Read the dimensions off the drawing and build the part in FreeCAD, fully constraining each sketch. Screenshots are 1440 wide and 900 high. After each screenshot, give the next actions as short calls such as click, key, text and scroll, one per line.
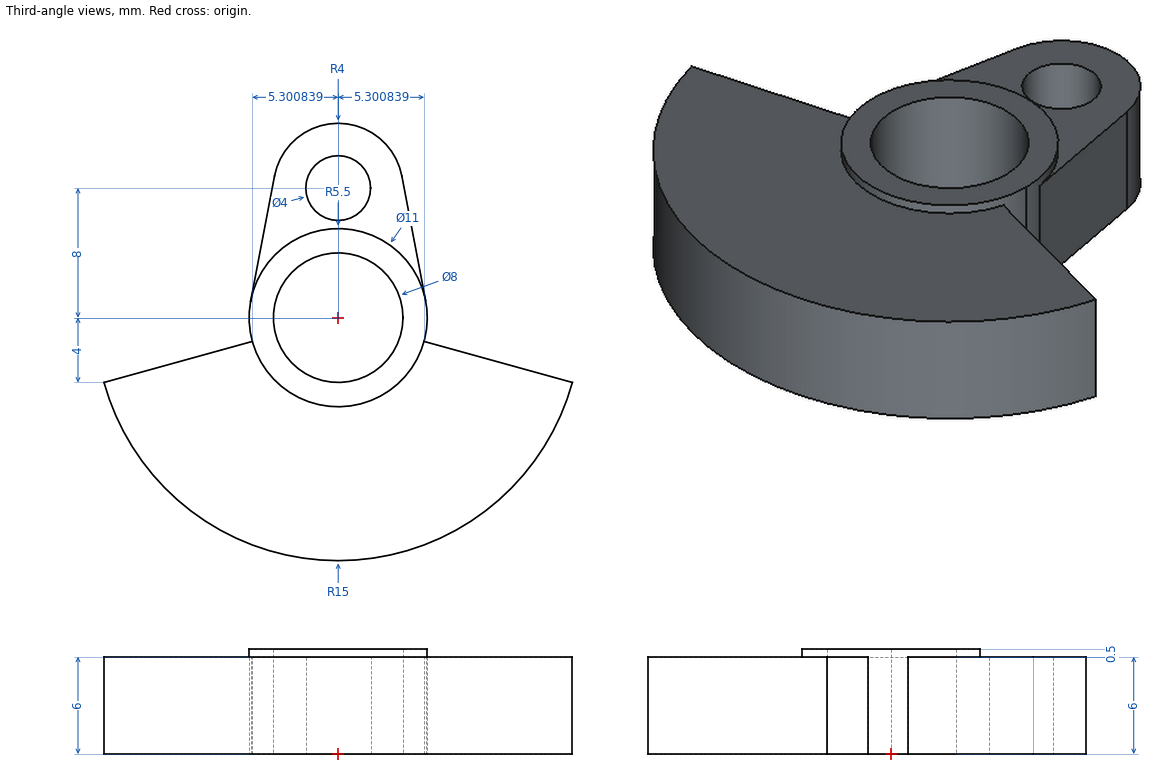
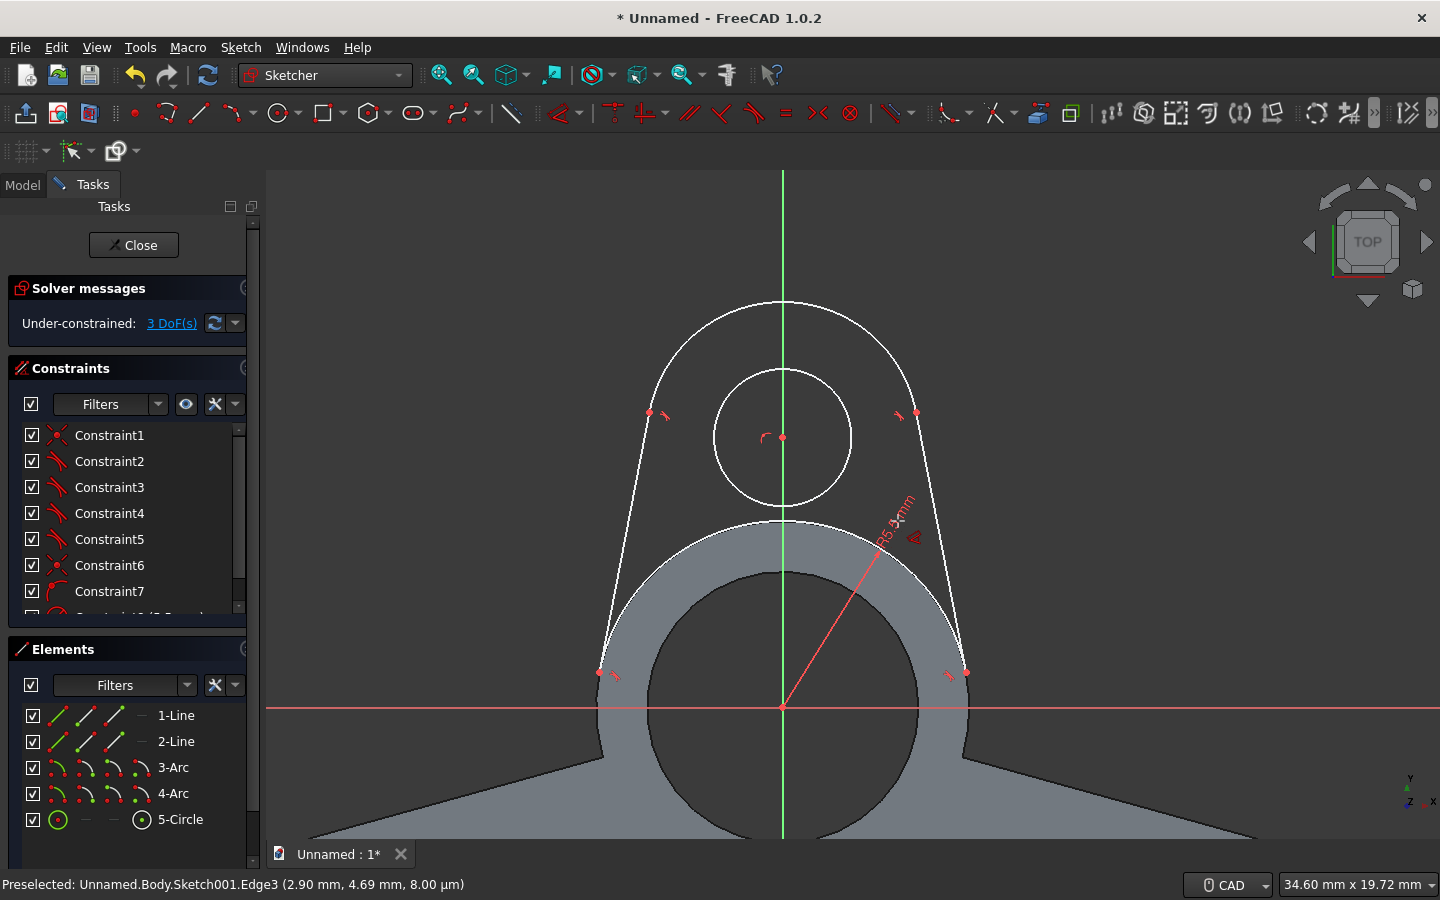
click(854, 322)
click(871, 295)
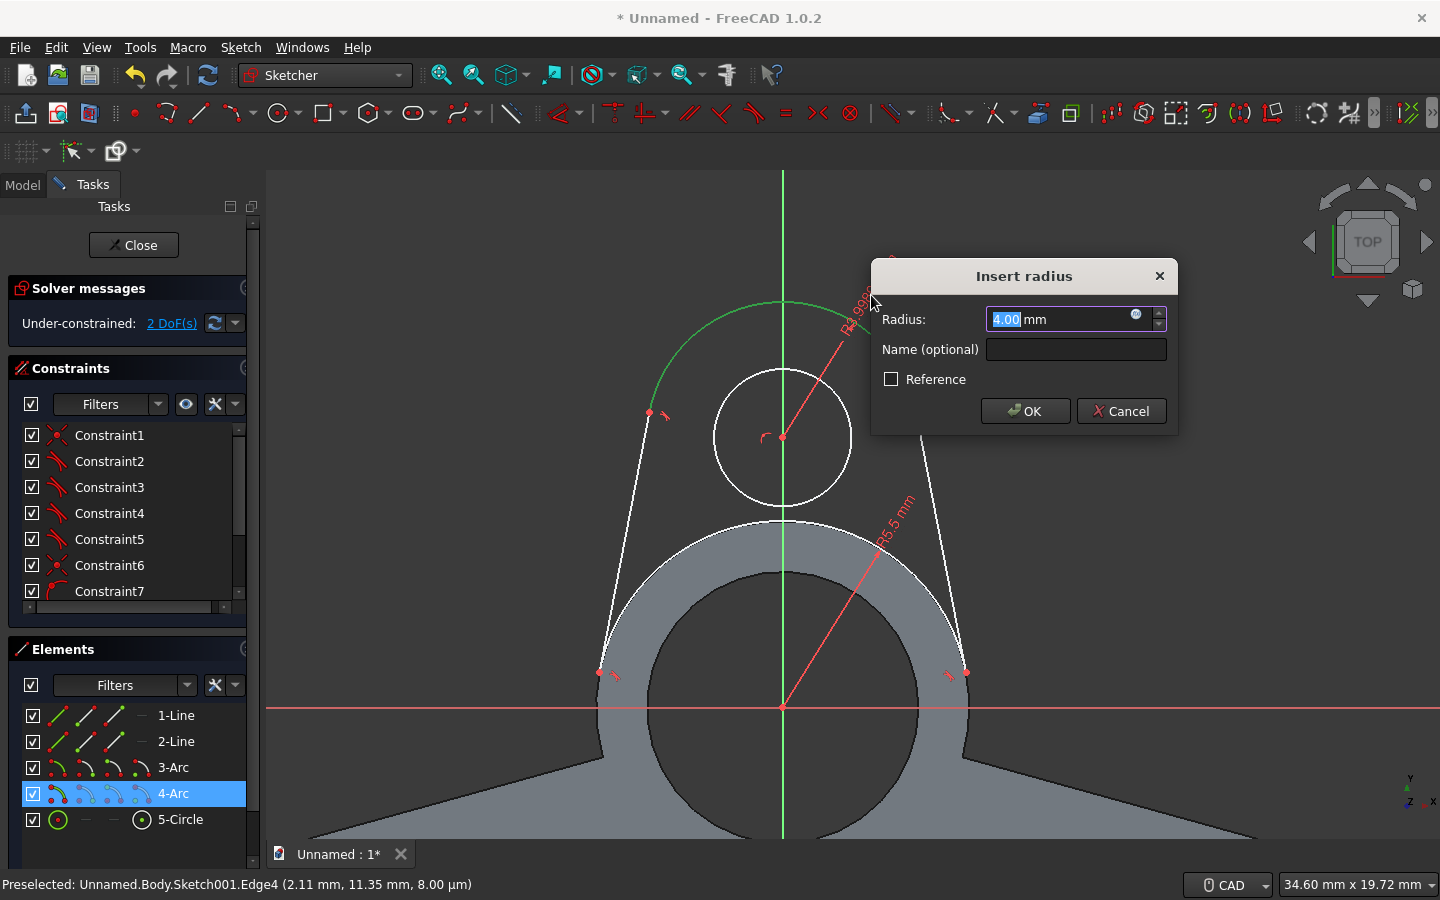
text(4)
key(Return)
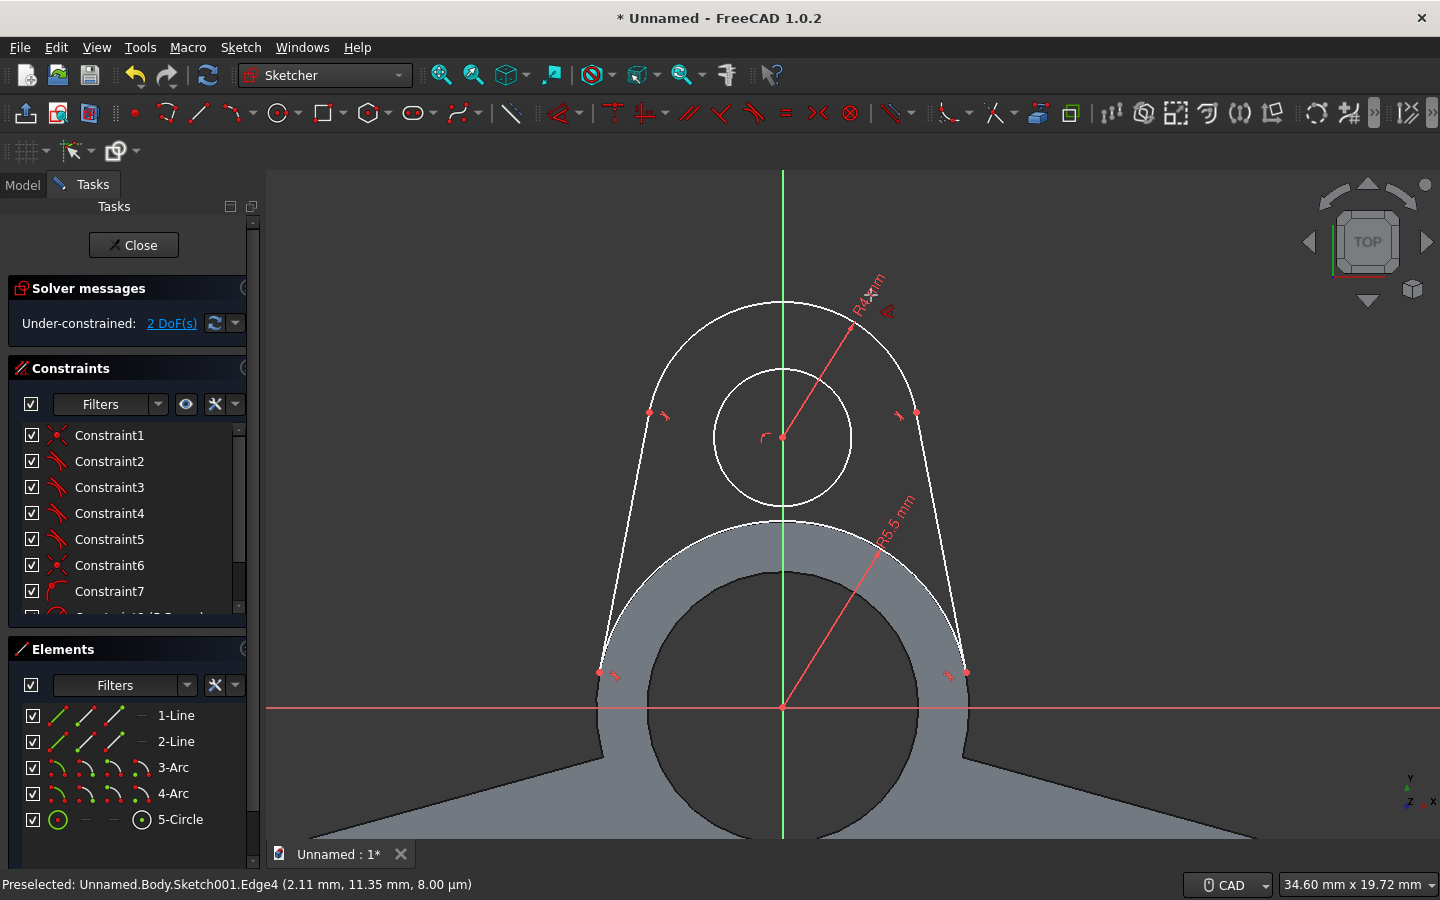
click(831, 389)
click(854, 366)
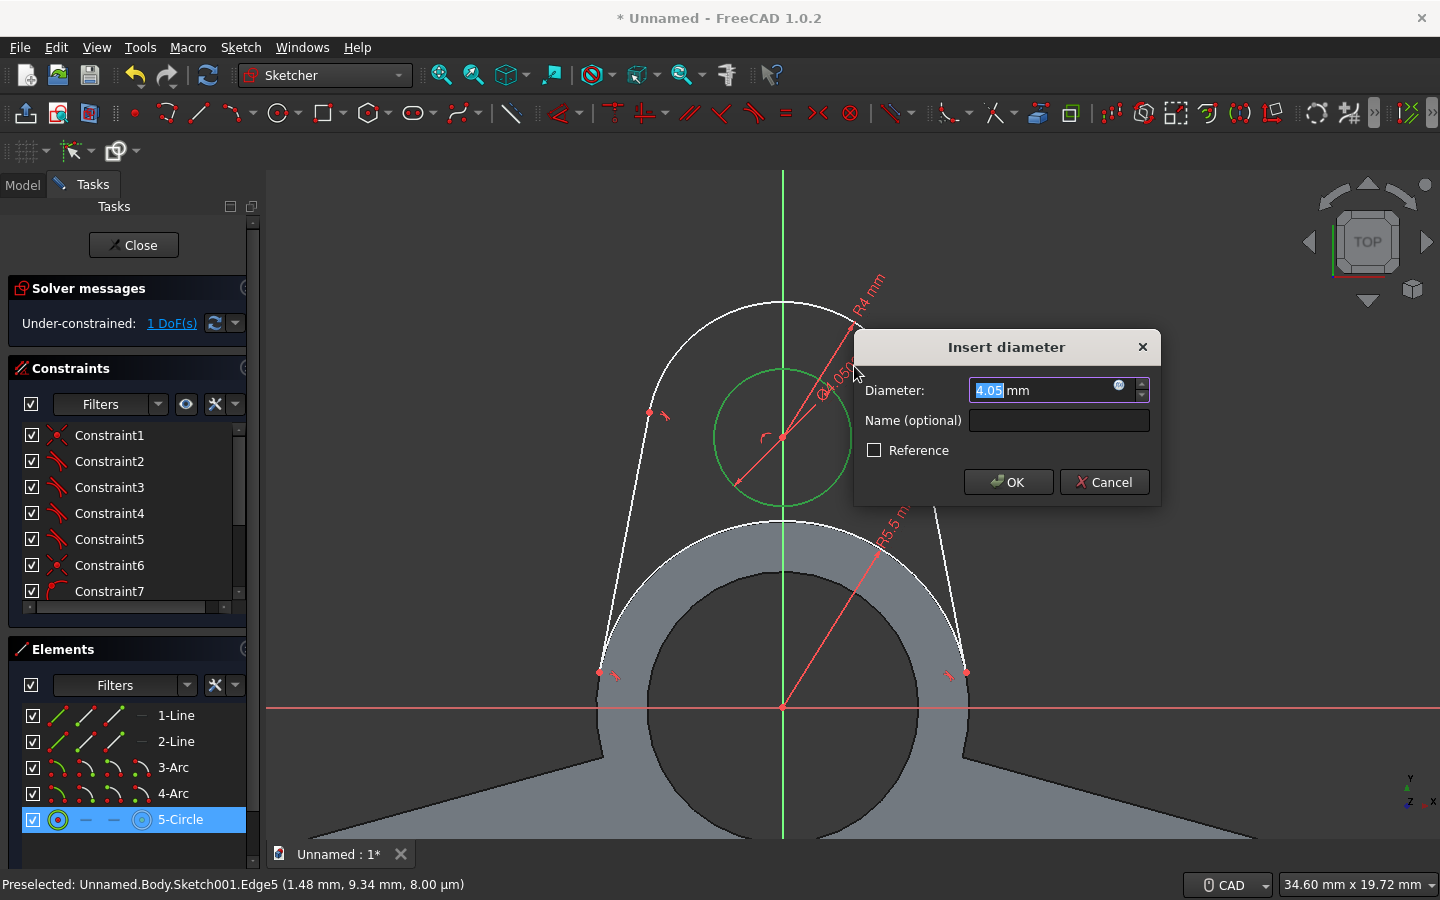
text(4)
key(Return)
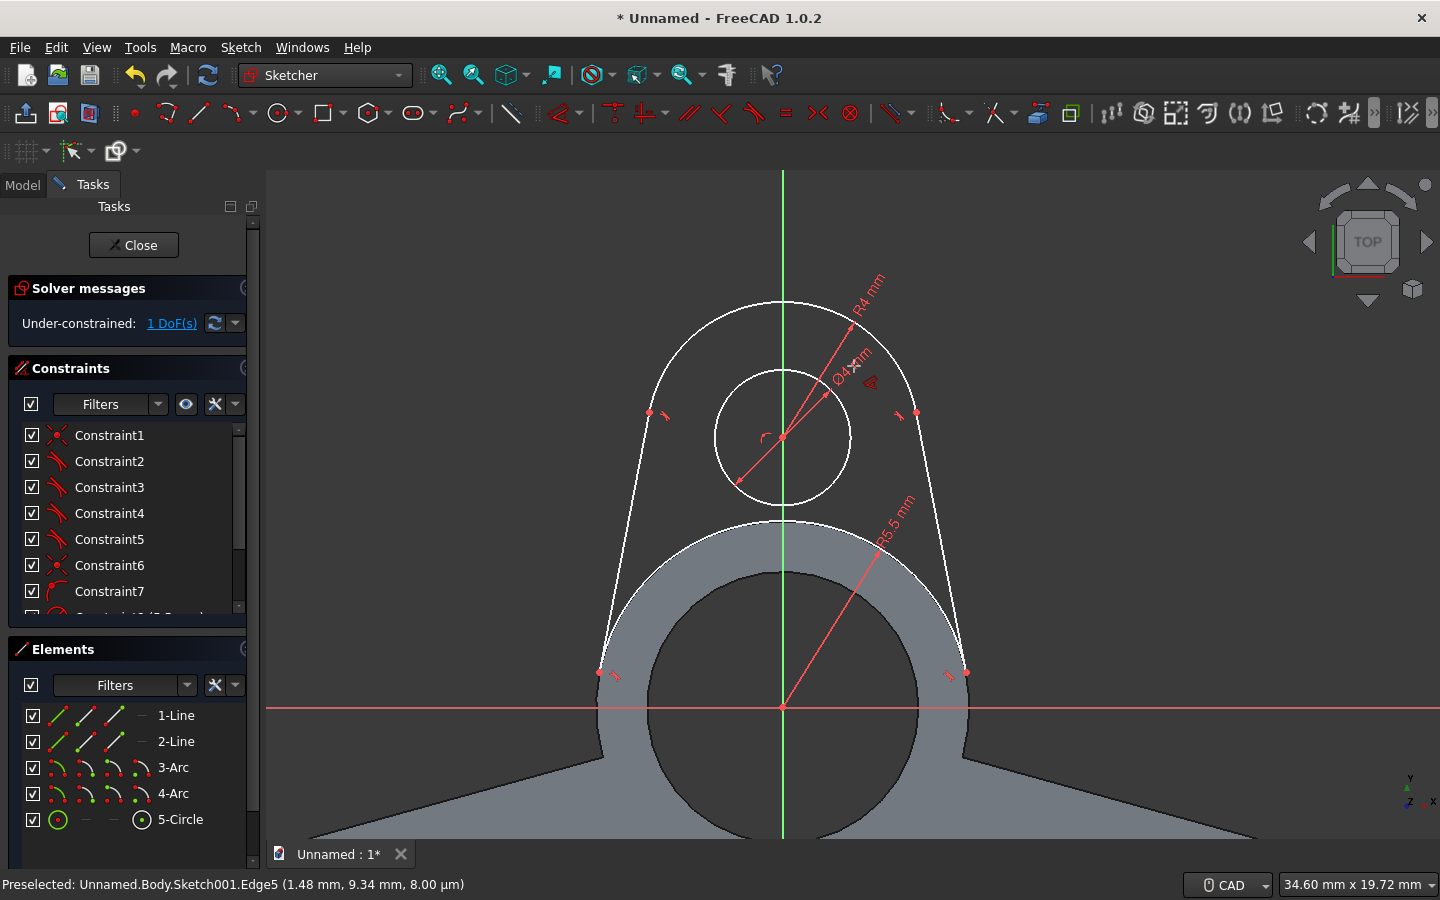
click(783, 438)
click(817, 573)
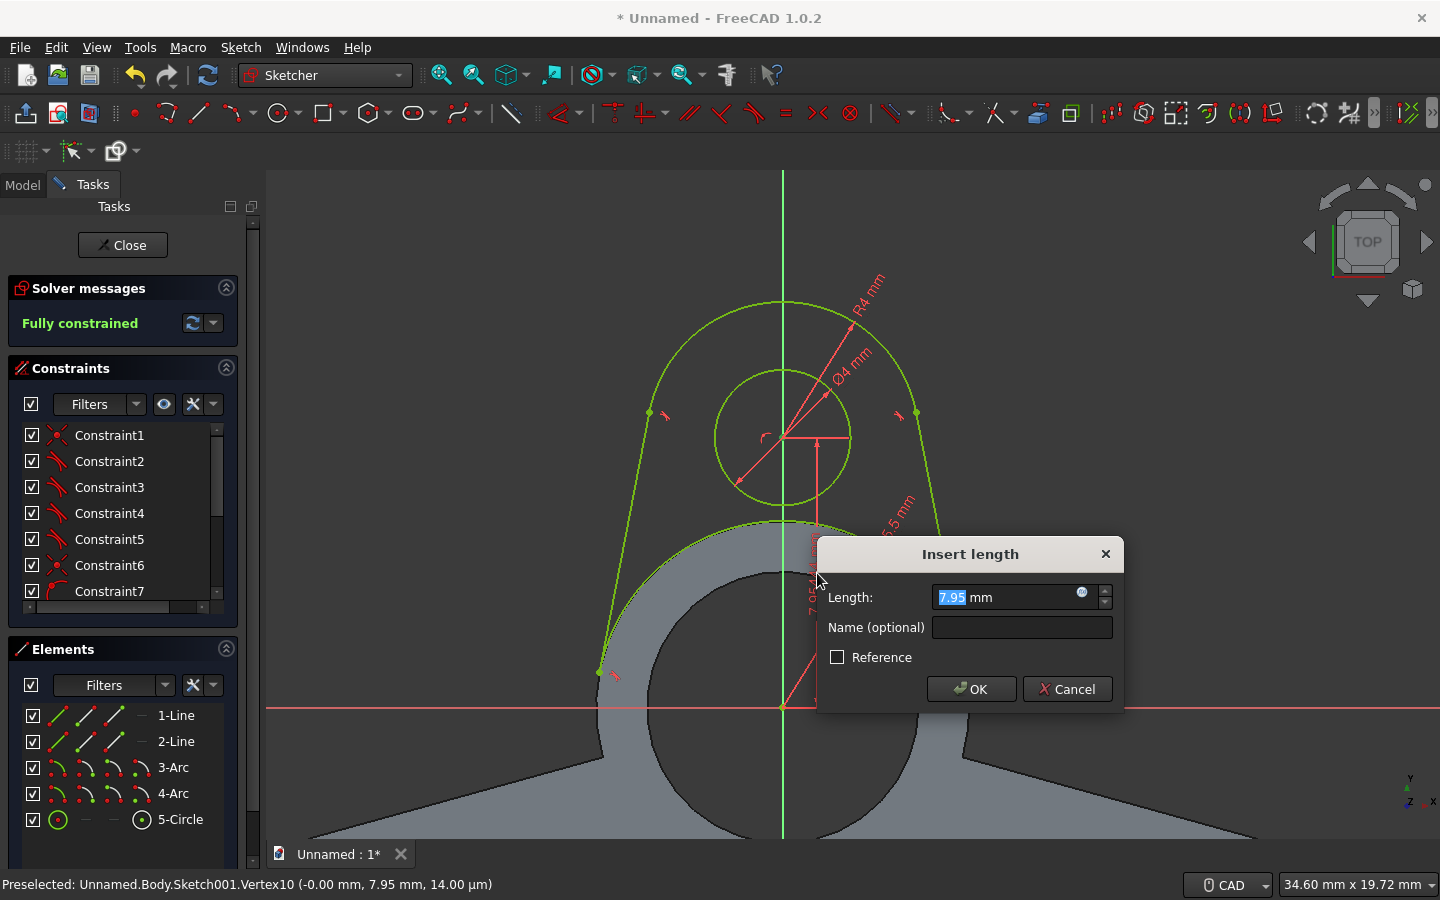
text(8)
key(Return)
key(Escape)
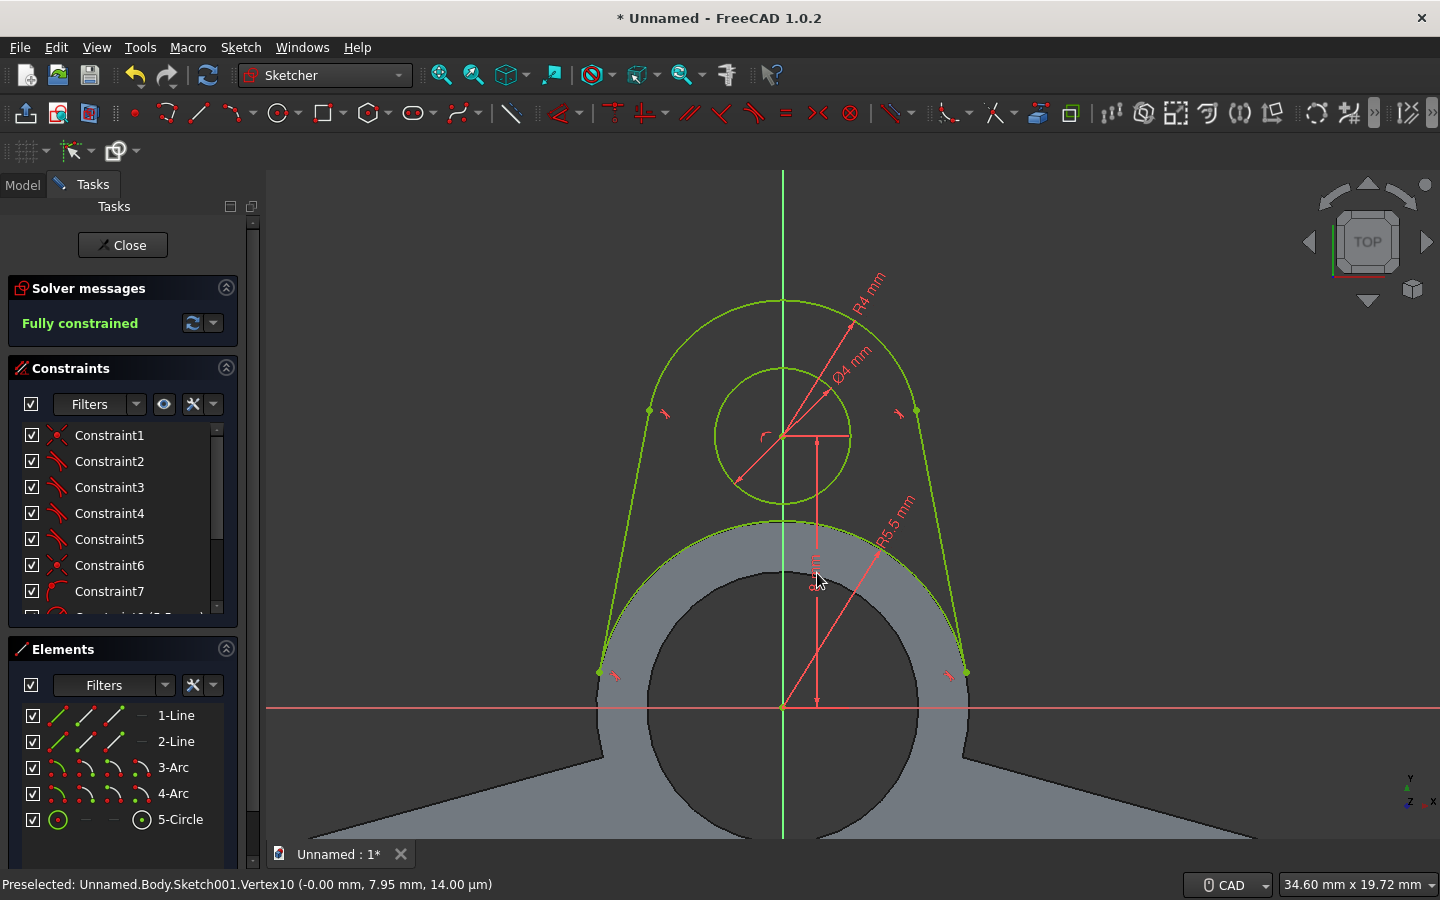
click(123, 245)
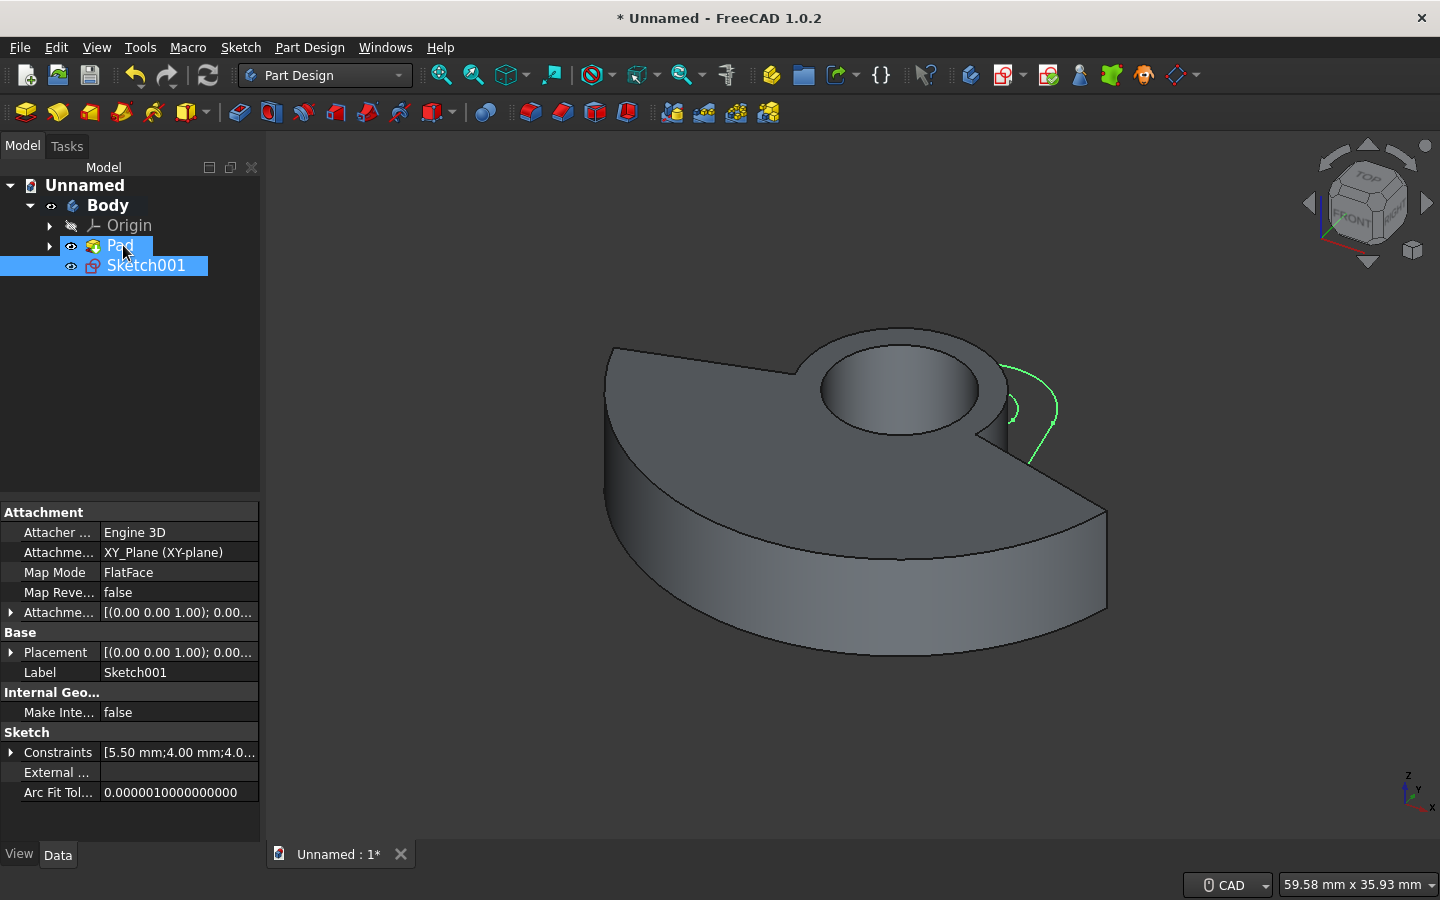
click(26, 112)